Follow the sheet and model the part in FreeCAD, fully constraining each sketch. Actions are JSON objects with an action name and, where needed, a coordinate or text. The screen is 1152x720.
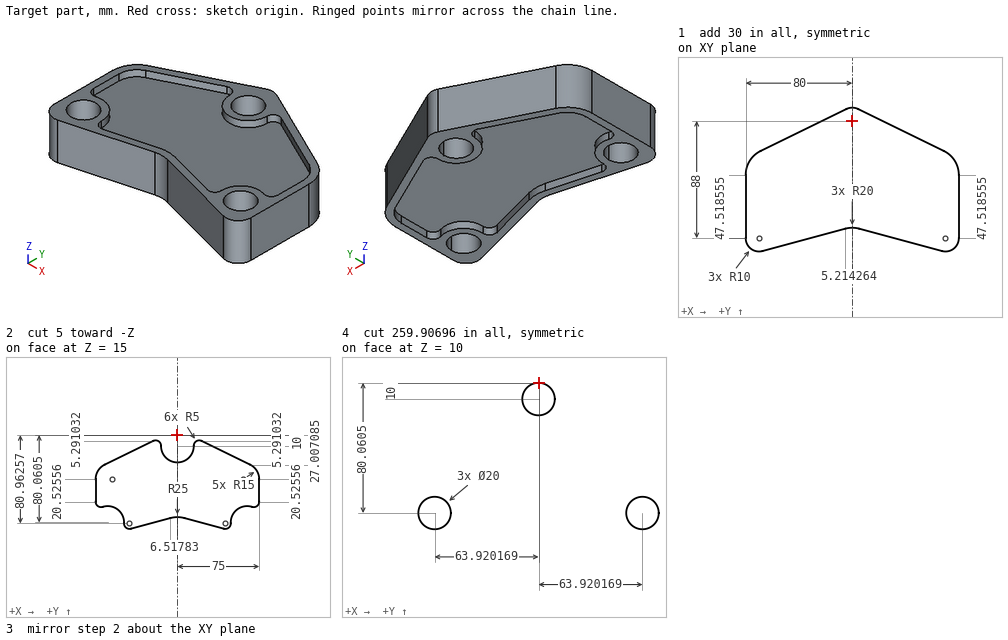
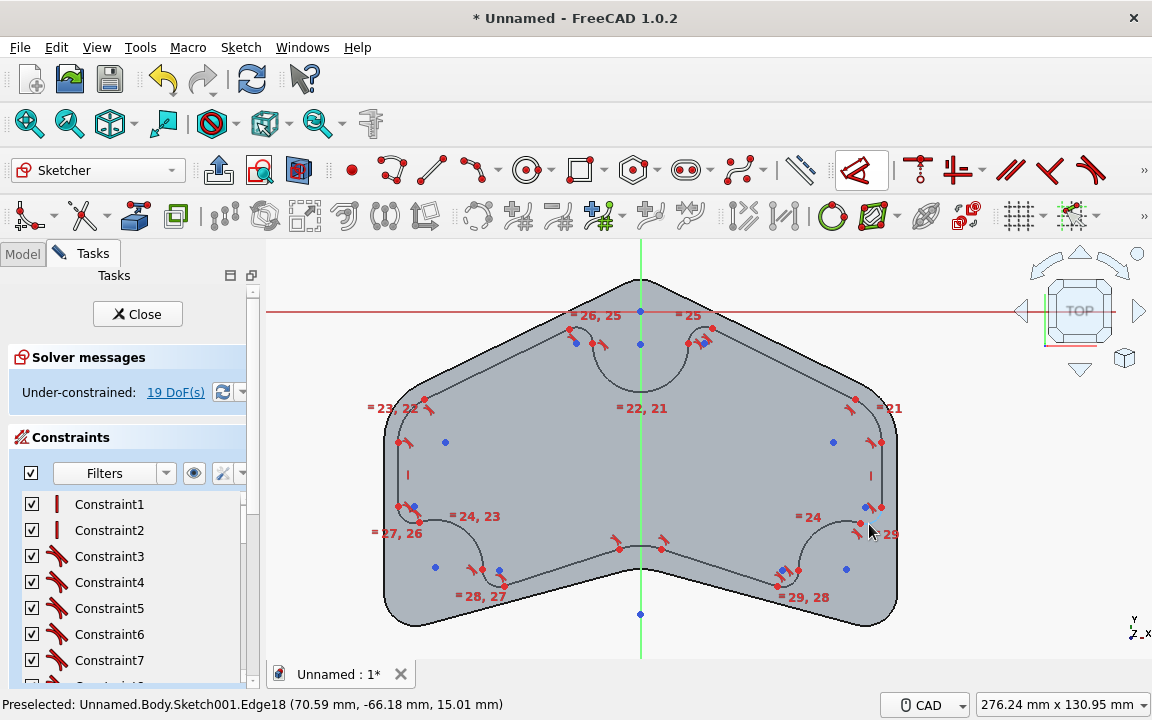
{"action": "left_click", "coordinate": [641, 344]}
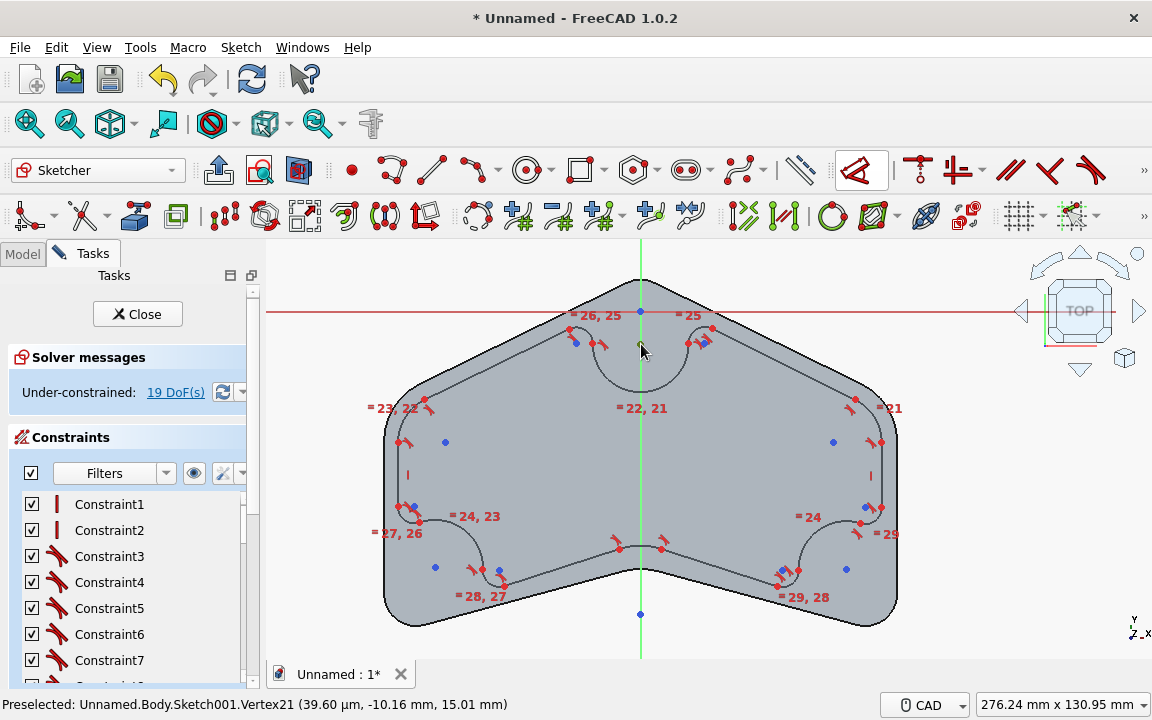
{"action": "left_click", "coordinate": [641, 605]}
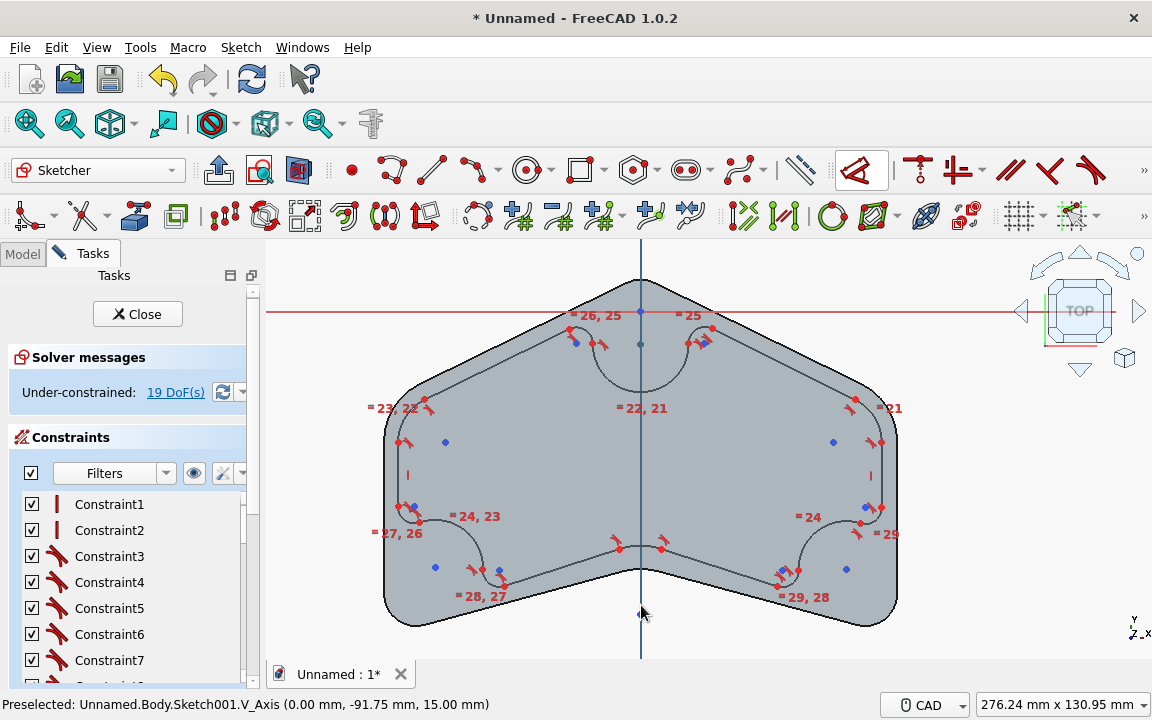
{"action": "key", "text": "c"}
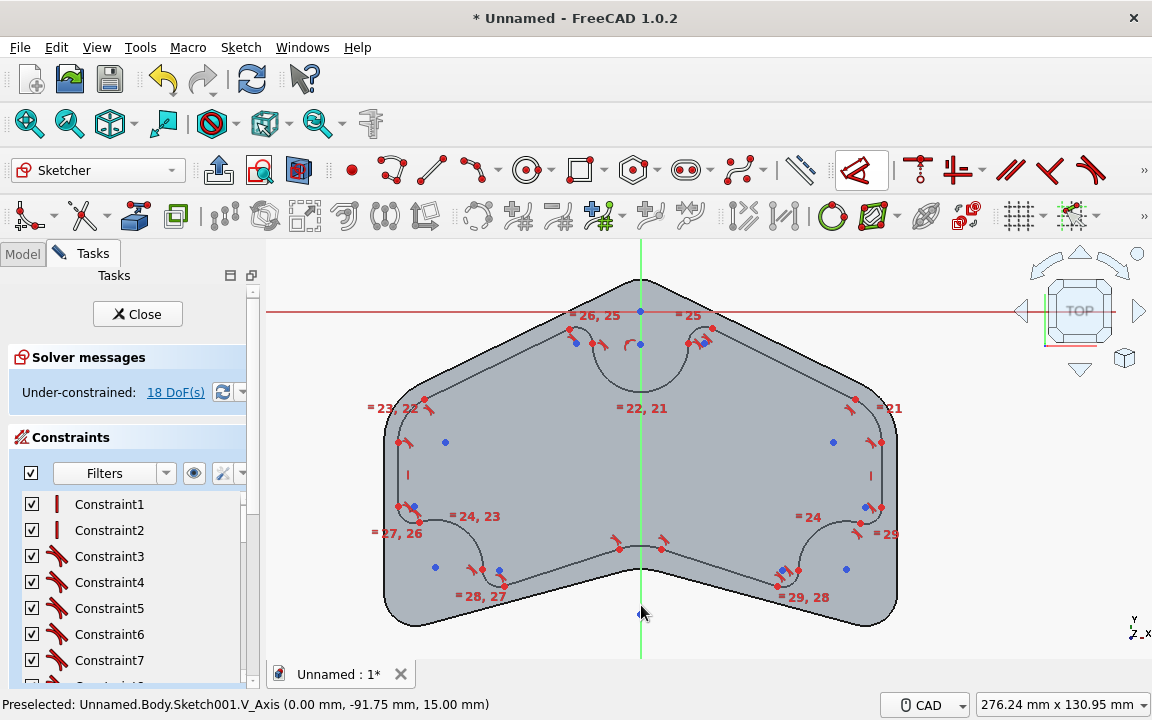
{"action": "left_click", "coordinate": [640, 614]}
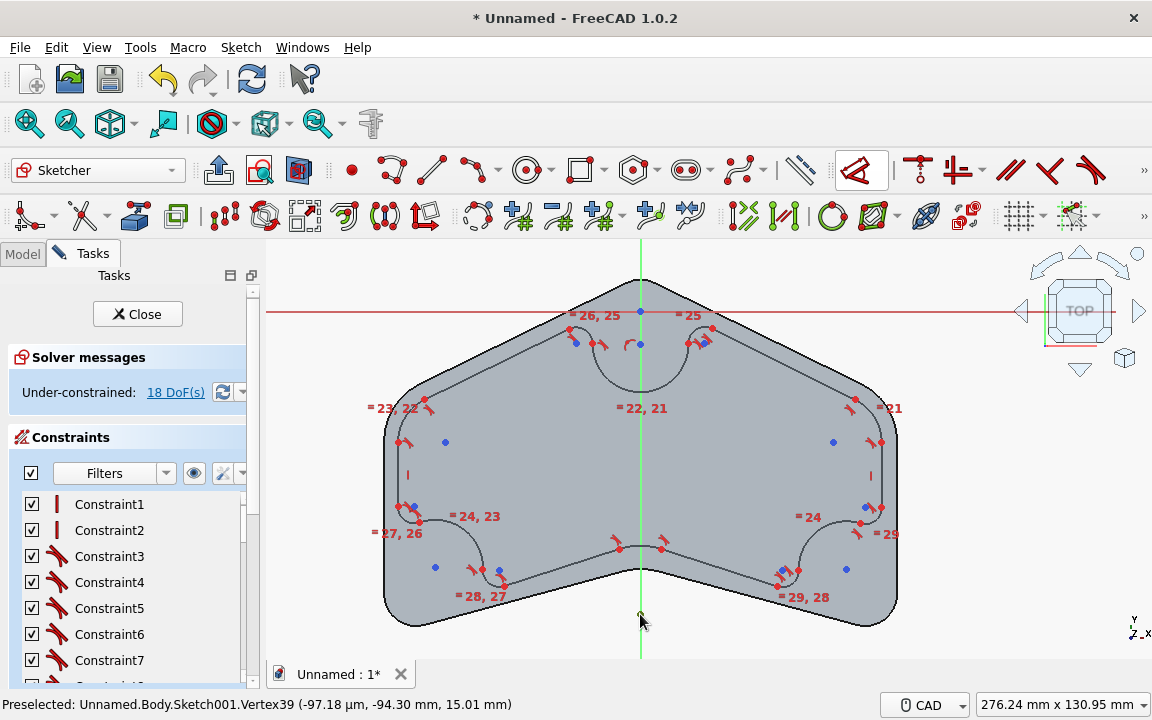
{"action": "left_click", "coordinate": [641, 605]}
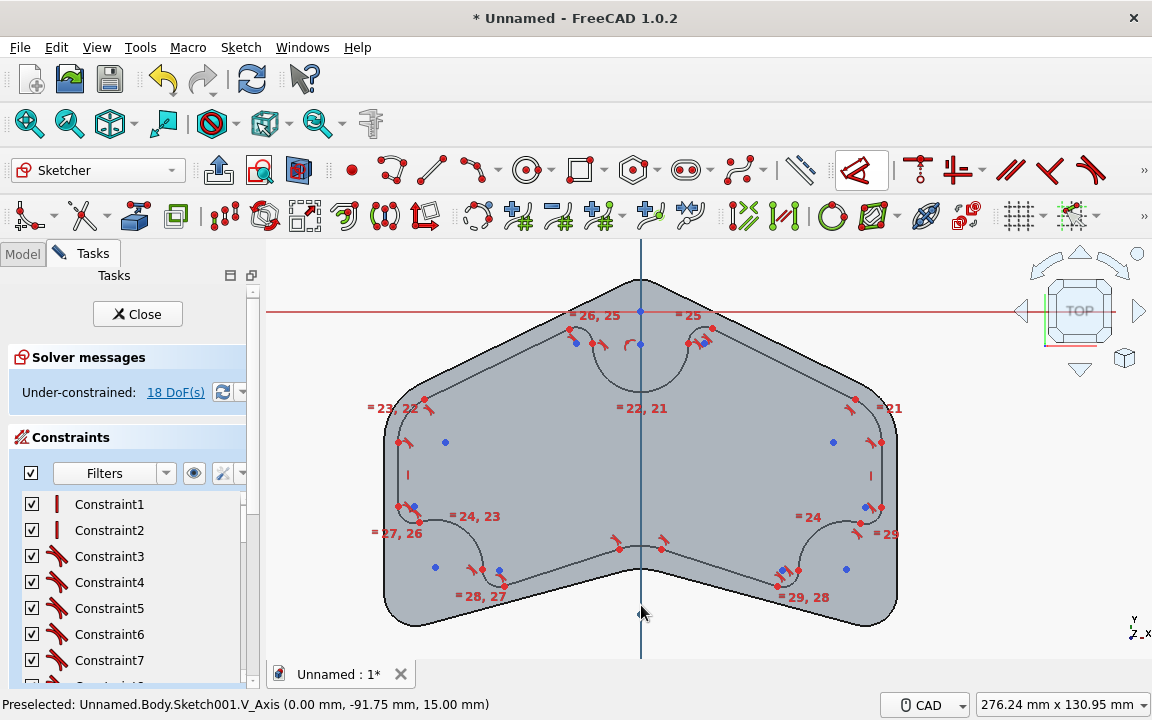
{"action": "left_click", "coordinate": [918, 170]}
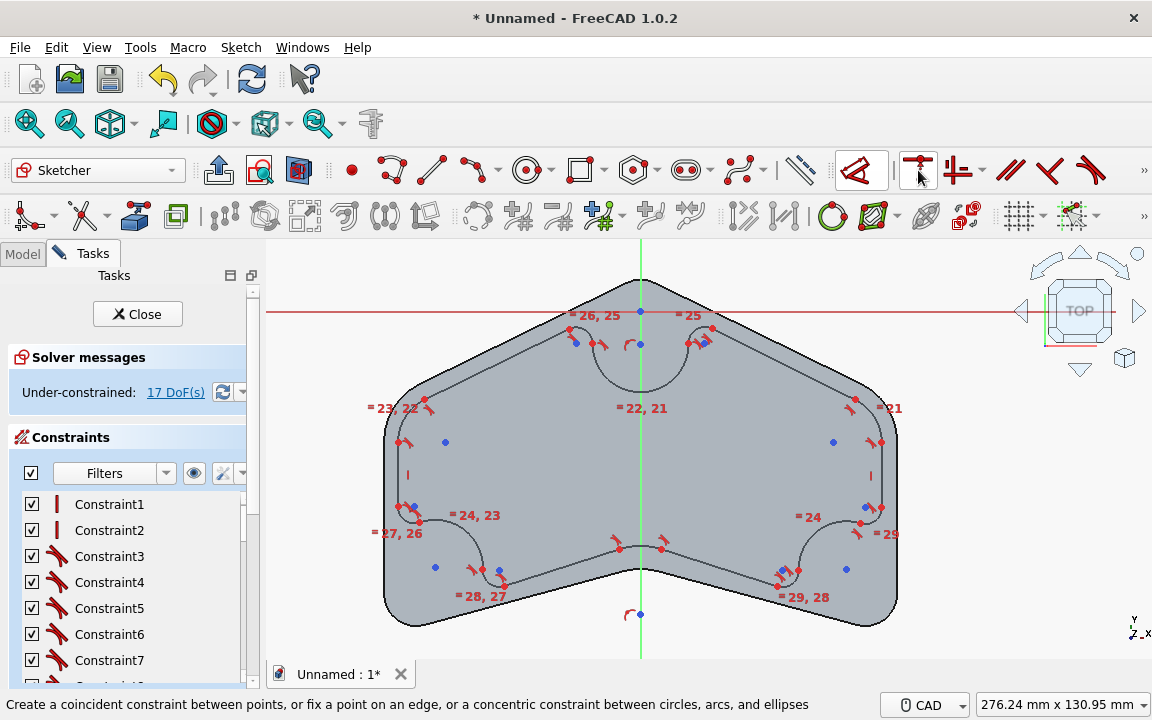
{"action": "left_click", "coordinate": [834, 443]}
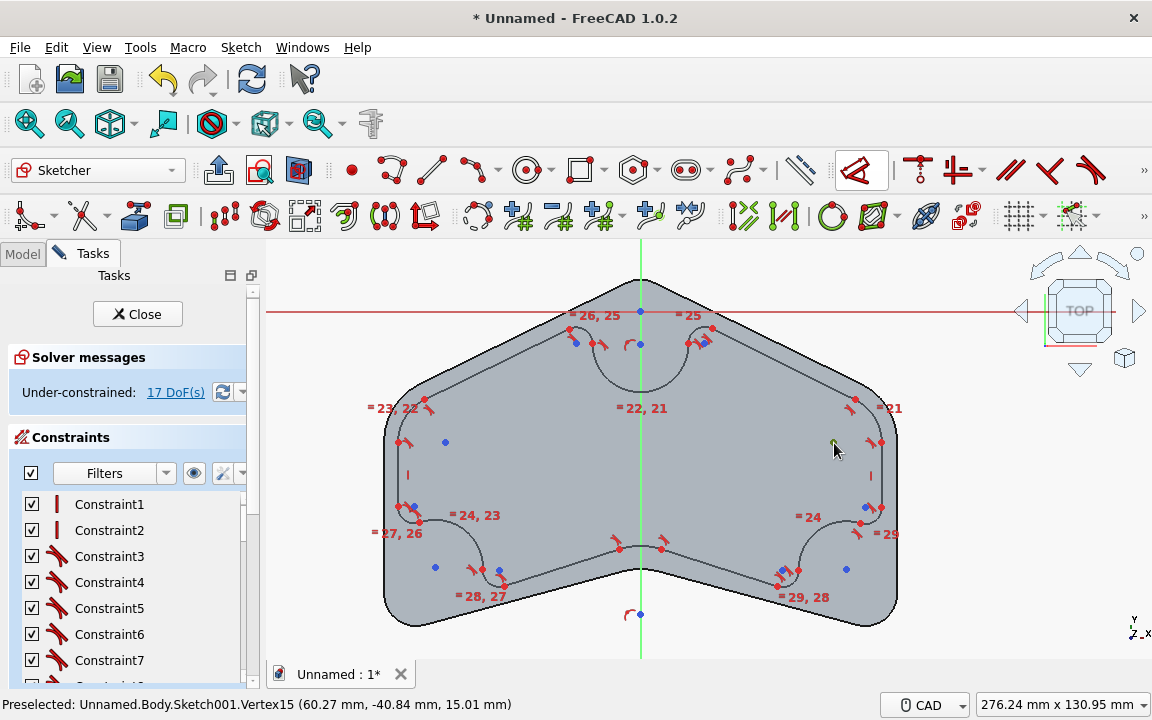
{"action": "left_click", "coordinate": [446, 443]}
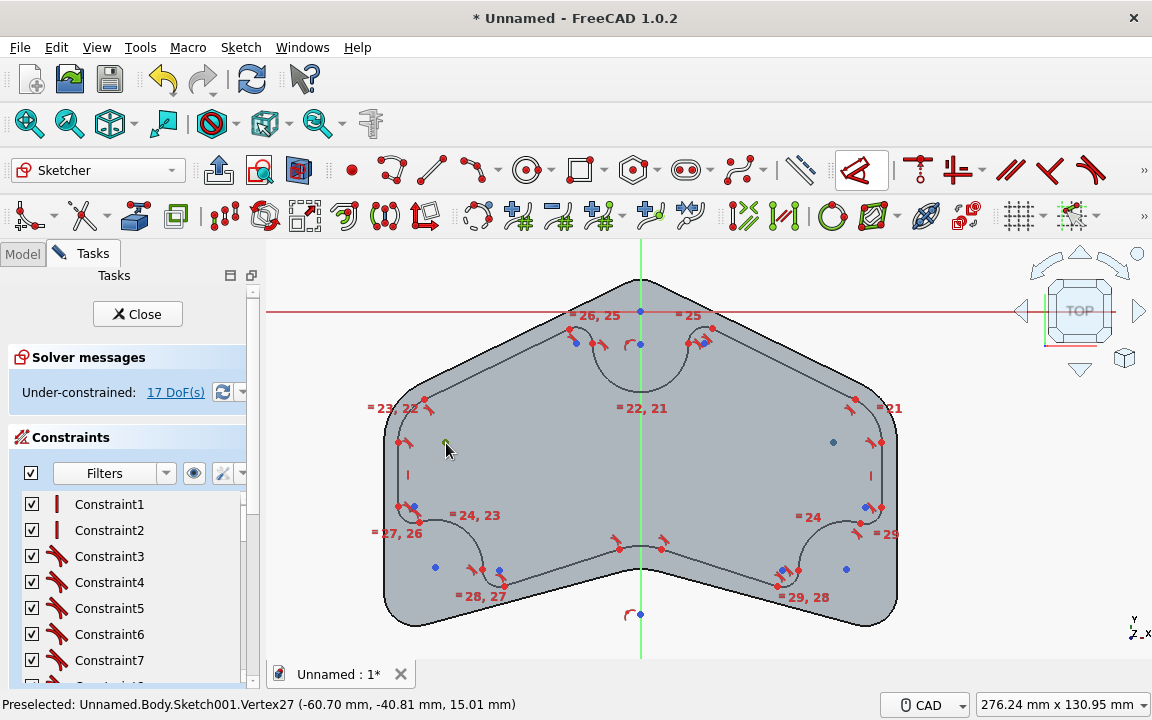
{"action": "left_click", "coordinate": [641, 605]}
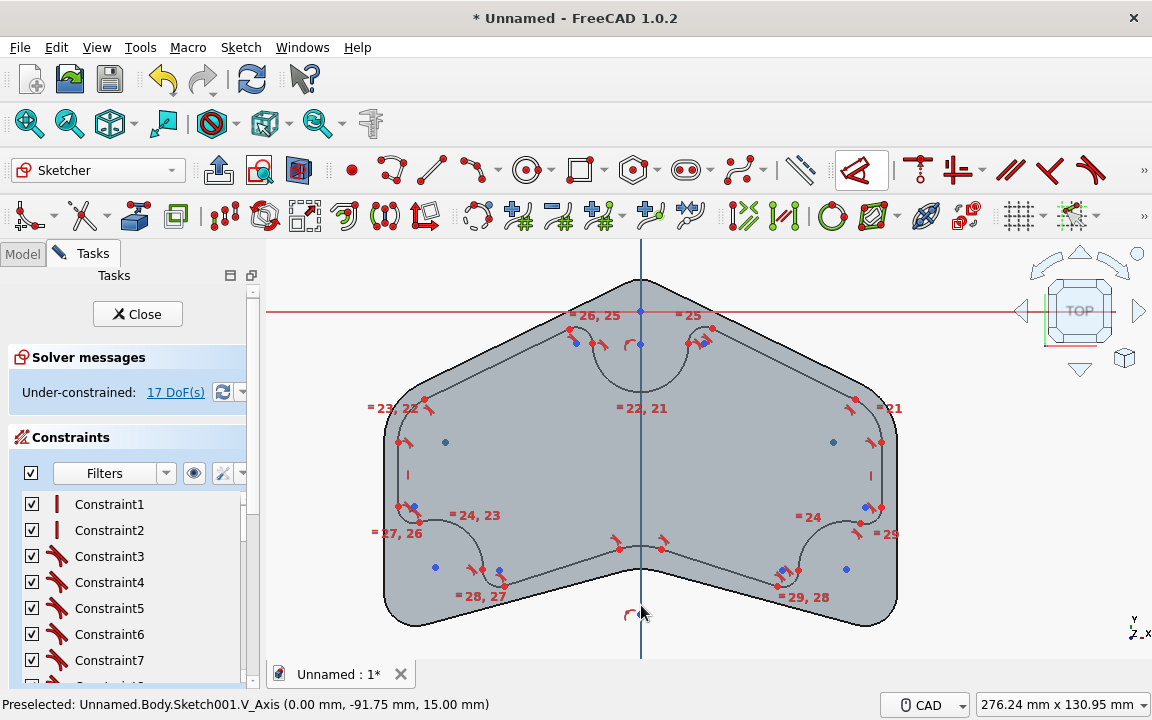
{"action": "key", "text": "s"}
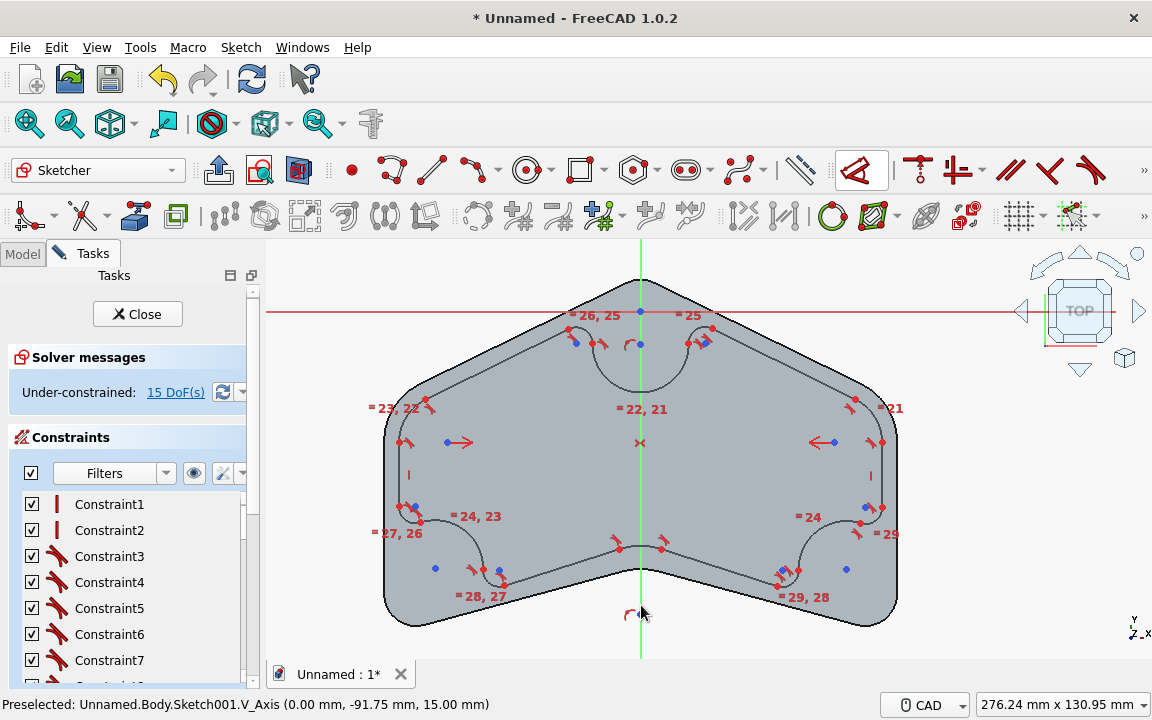
{"action": "left_click", "coordinate": [499, 570]}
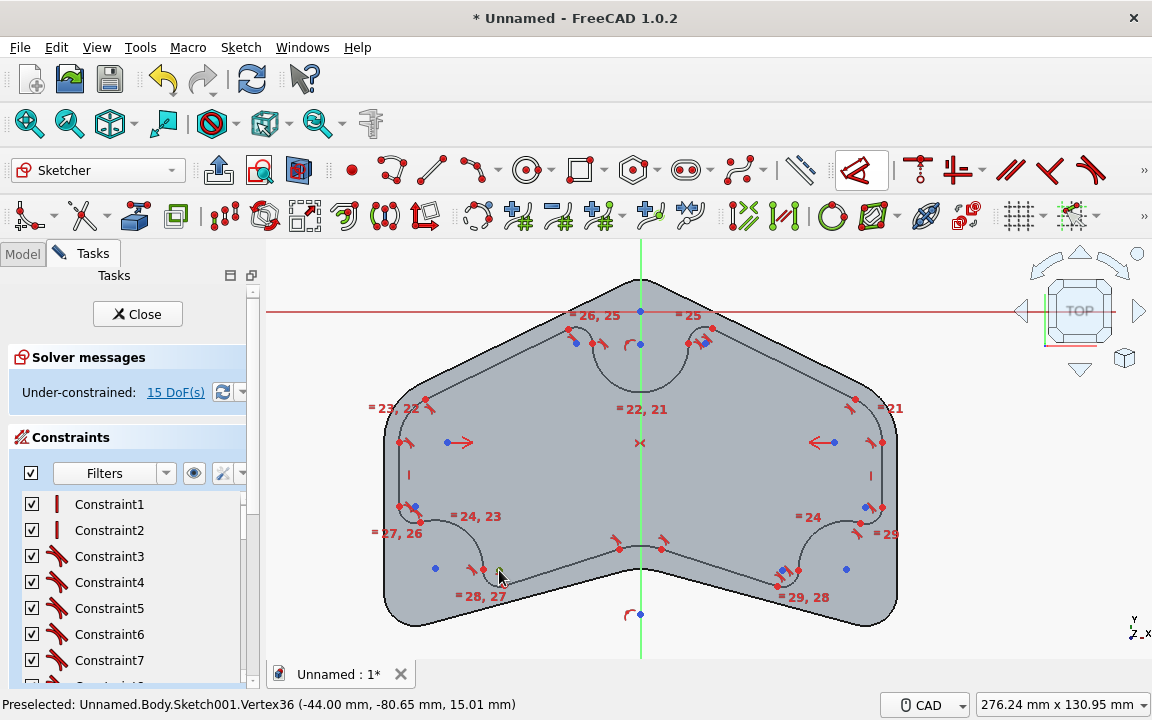
{"action": "left_click", "coordinate": [782, 571]}